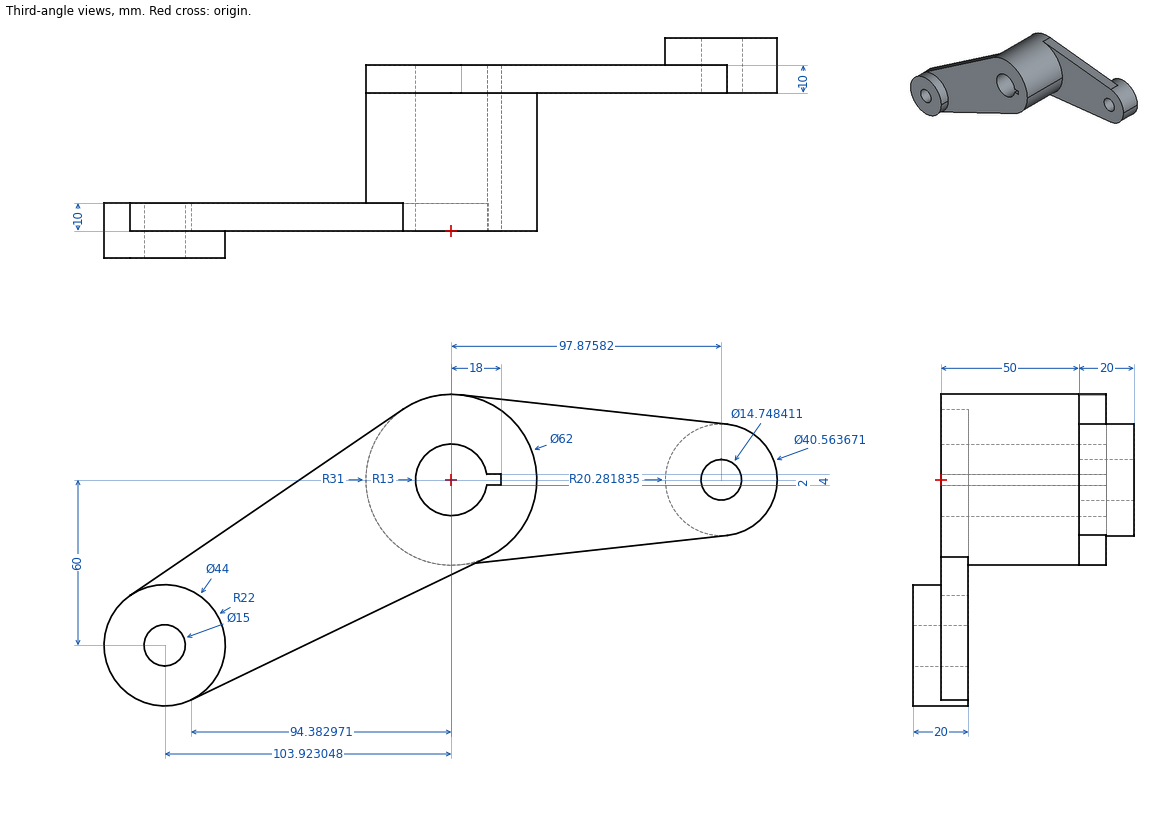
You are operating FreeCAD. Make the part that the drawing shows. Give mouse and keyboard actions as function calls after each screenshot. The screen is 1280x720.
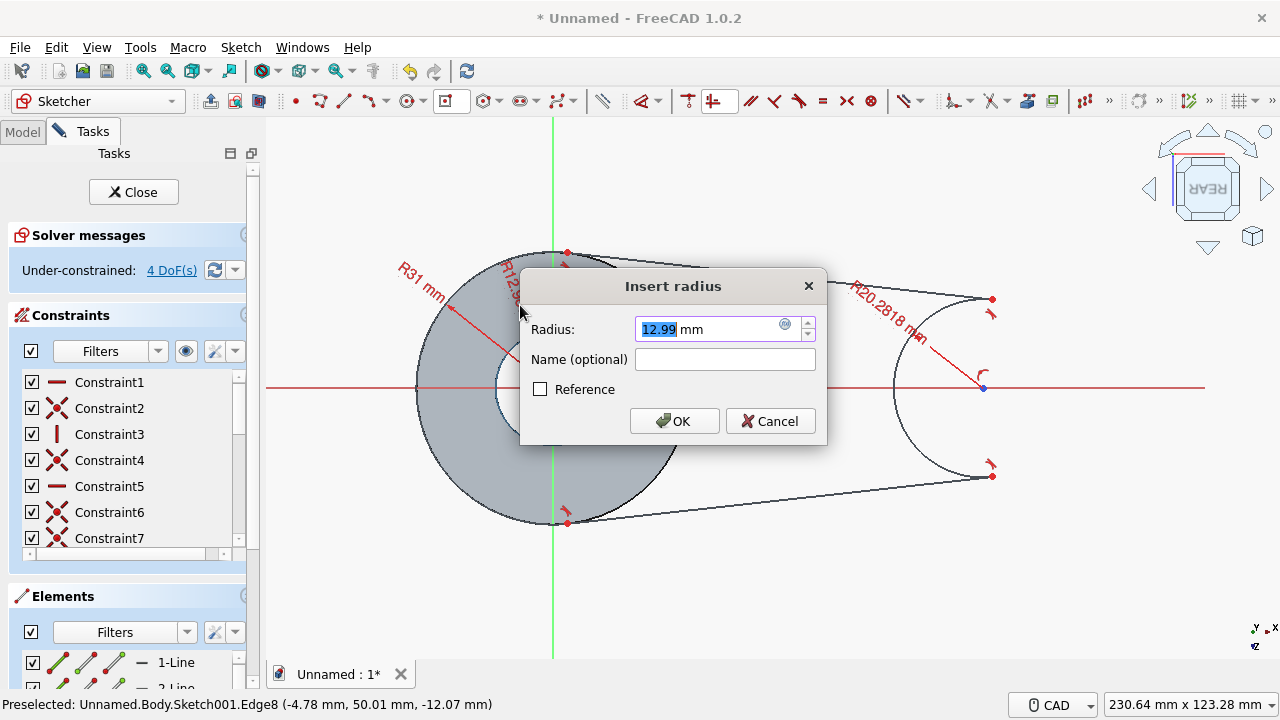
text(13)
key(Return)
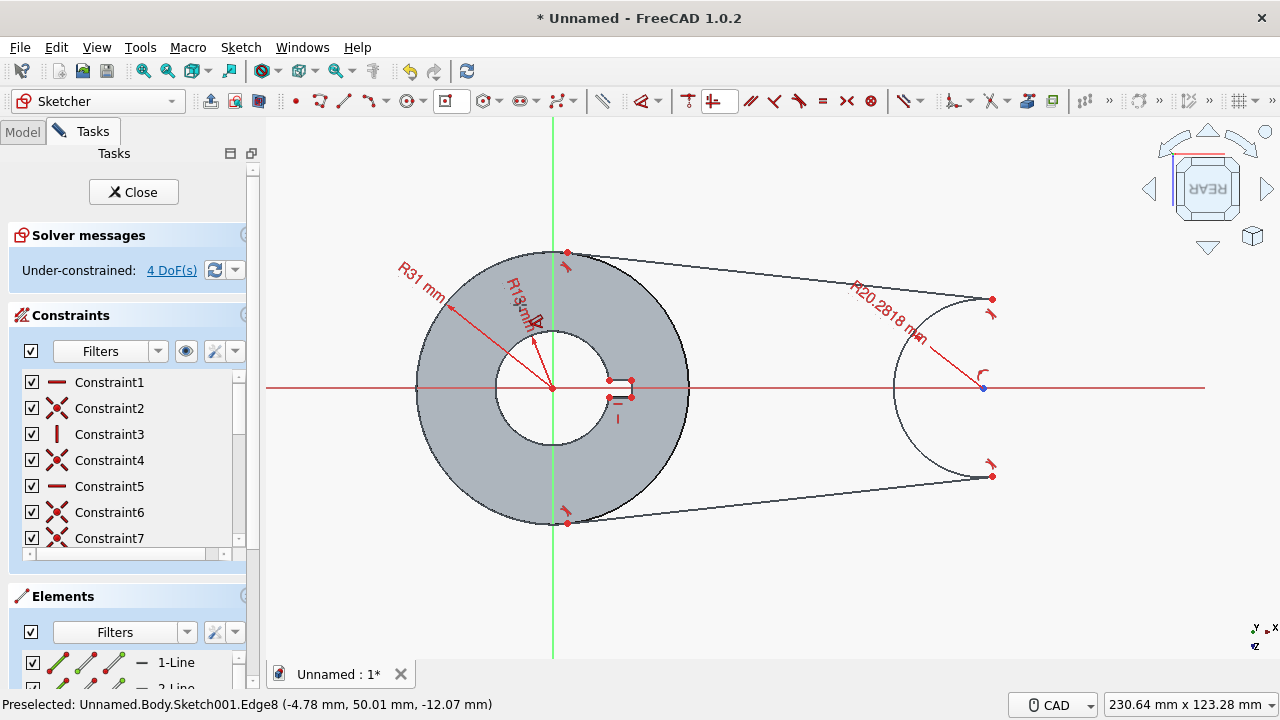
scroll(632, 389, up, 5)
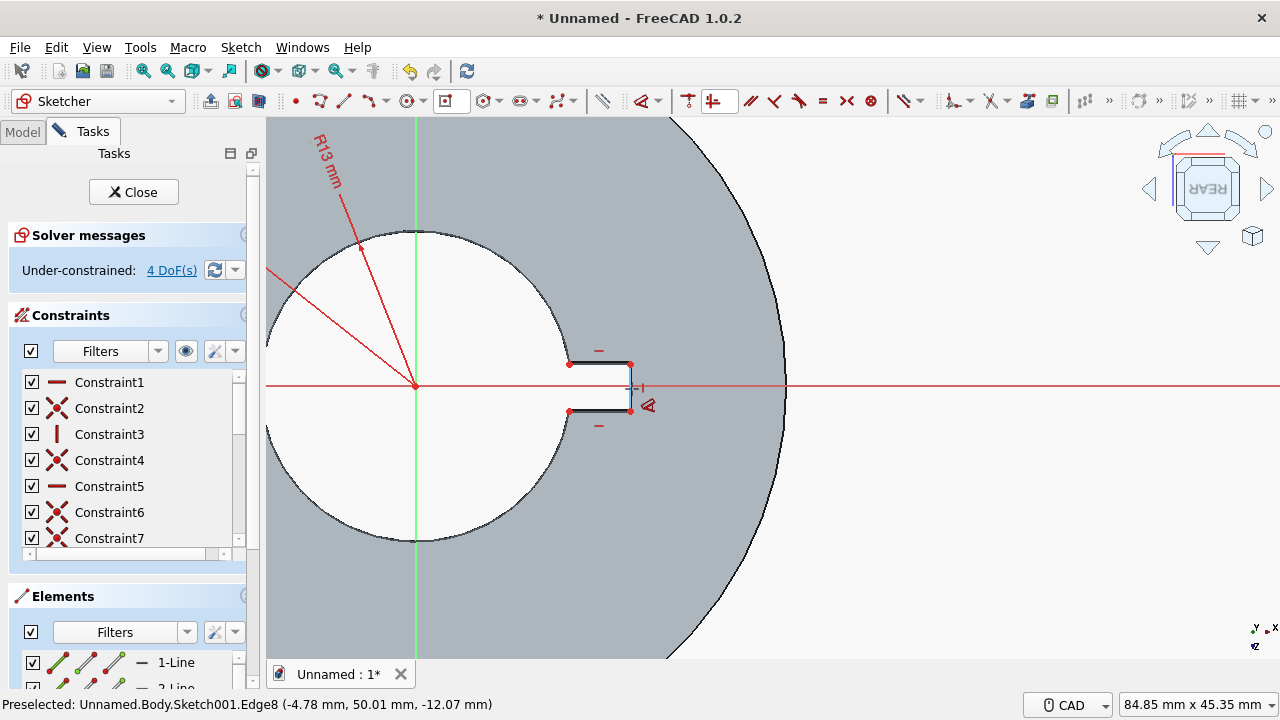
click(630, 388)
click(664, 371)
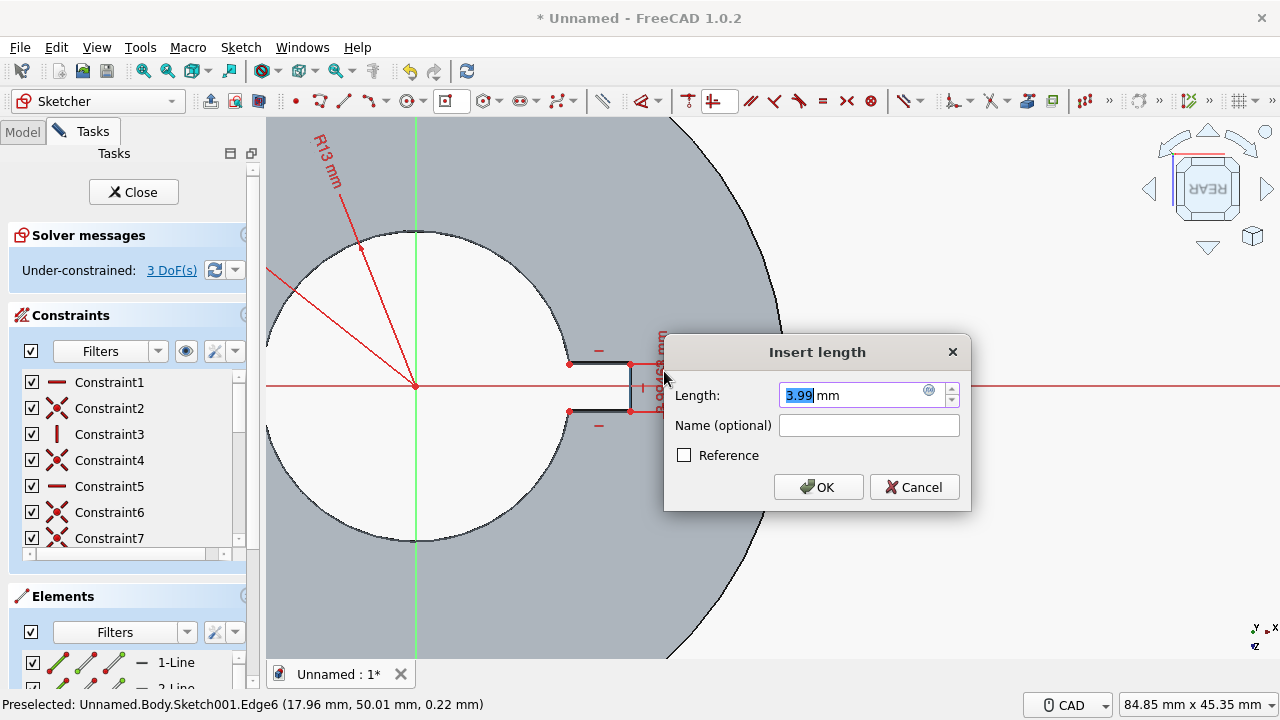
text(4)
key(Return)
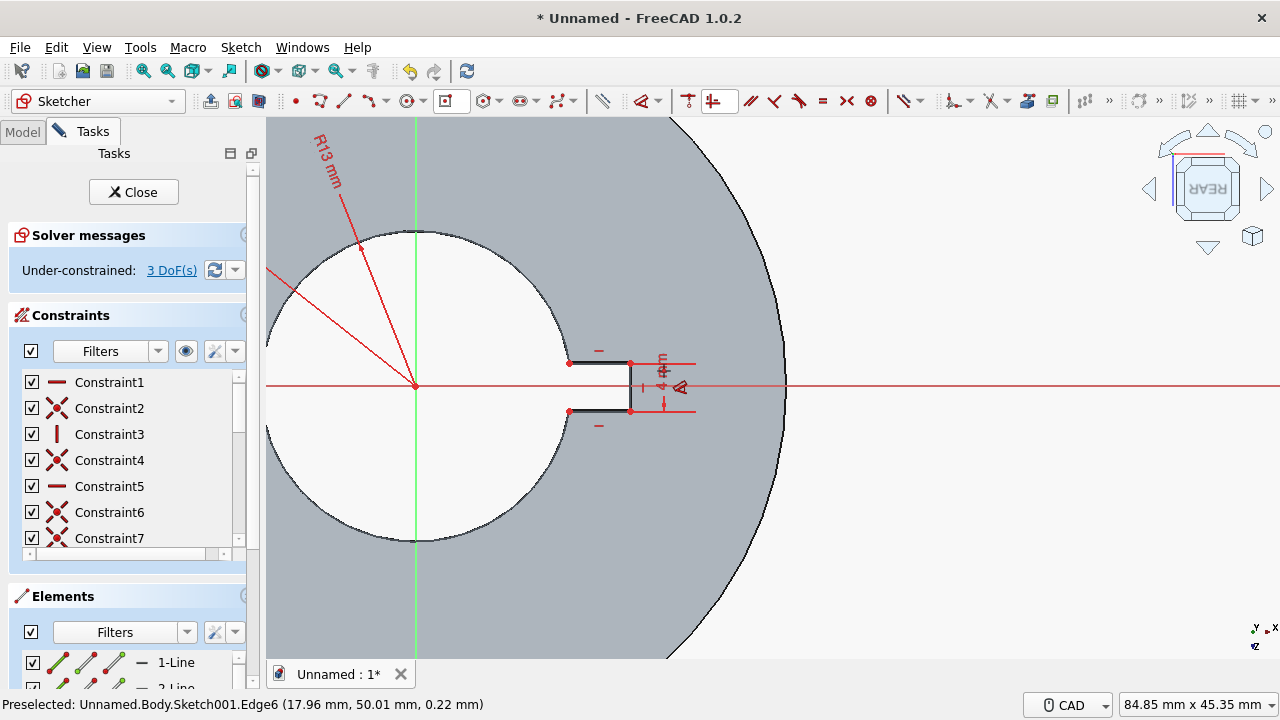
scroll(569, 364, up, 3)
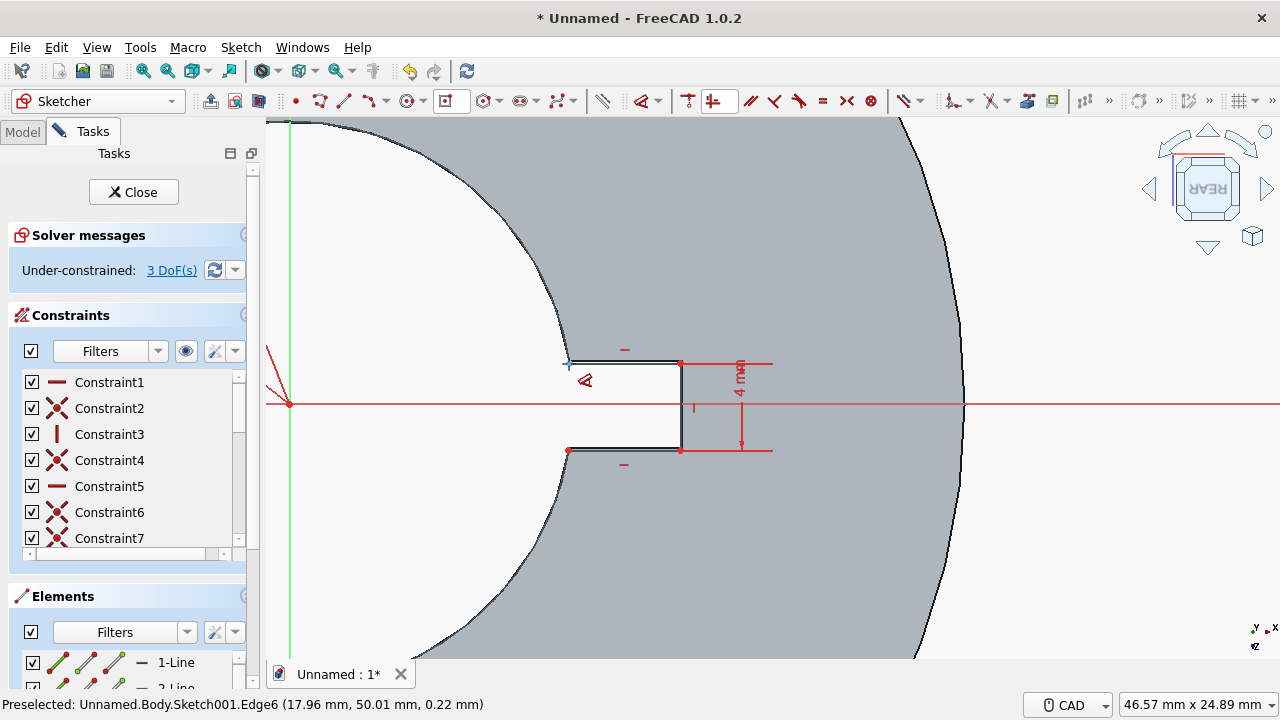
click(570, 364)
click(604, 384)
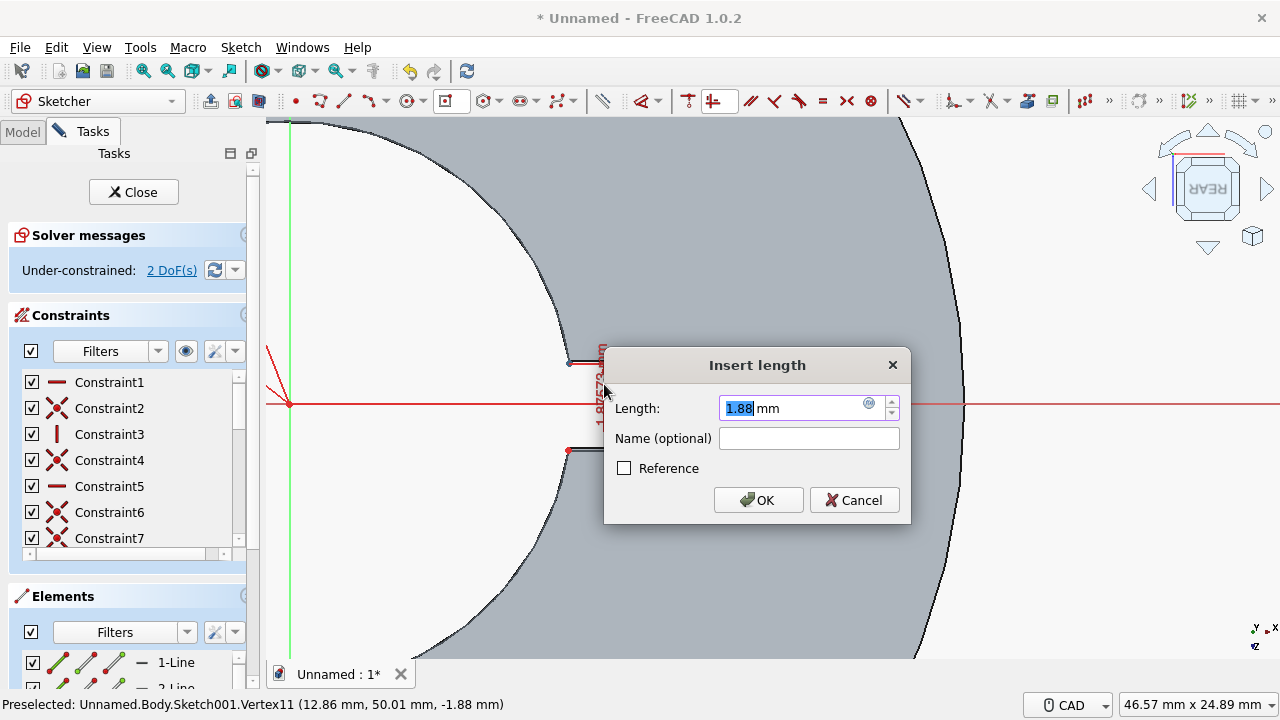
text(2)
key(Return)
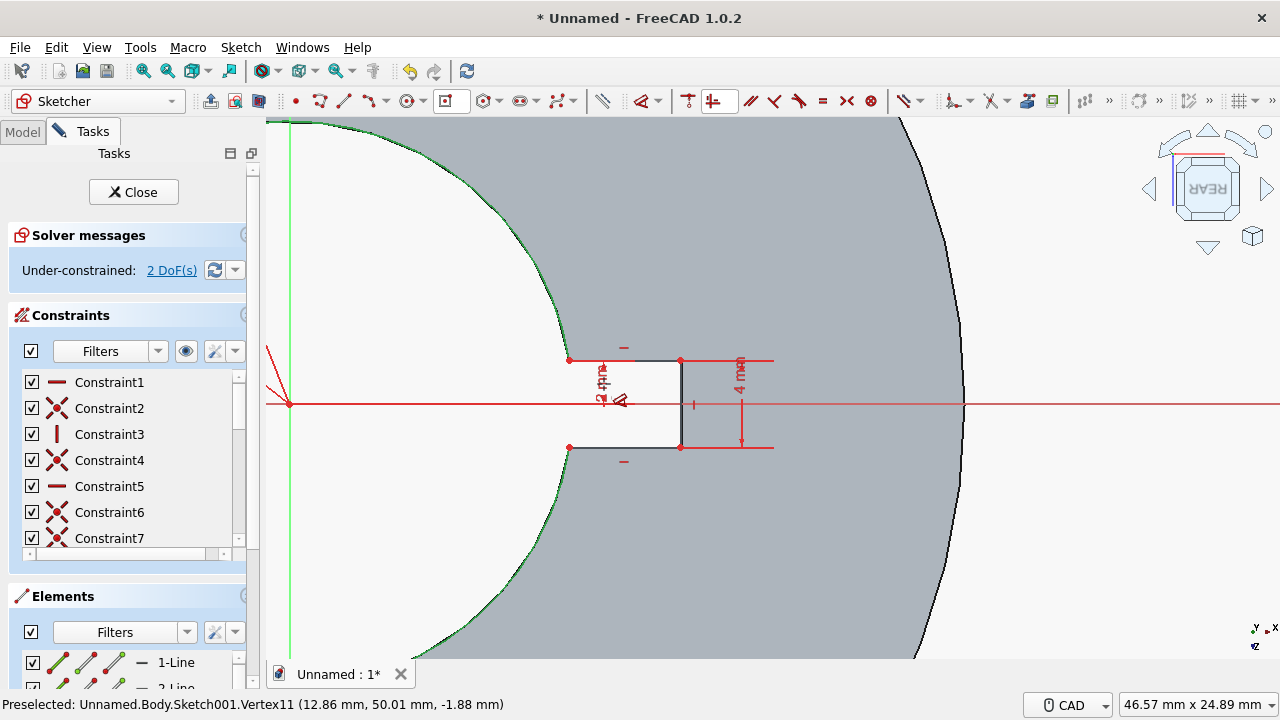
scroll(619, 384, down, 8)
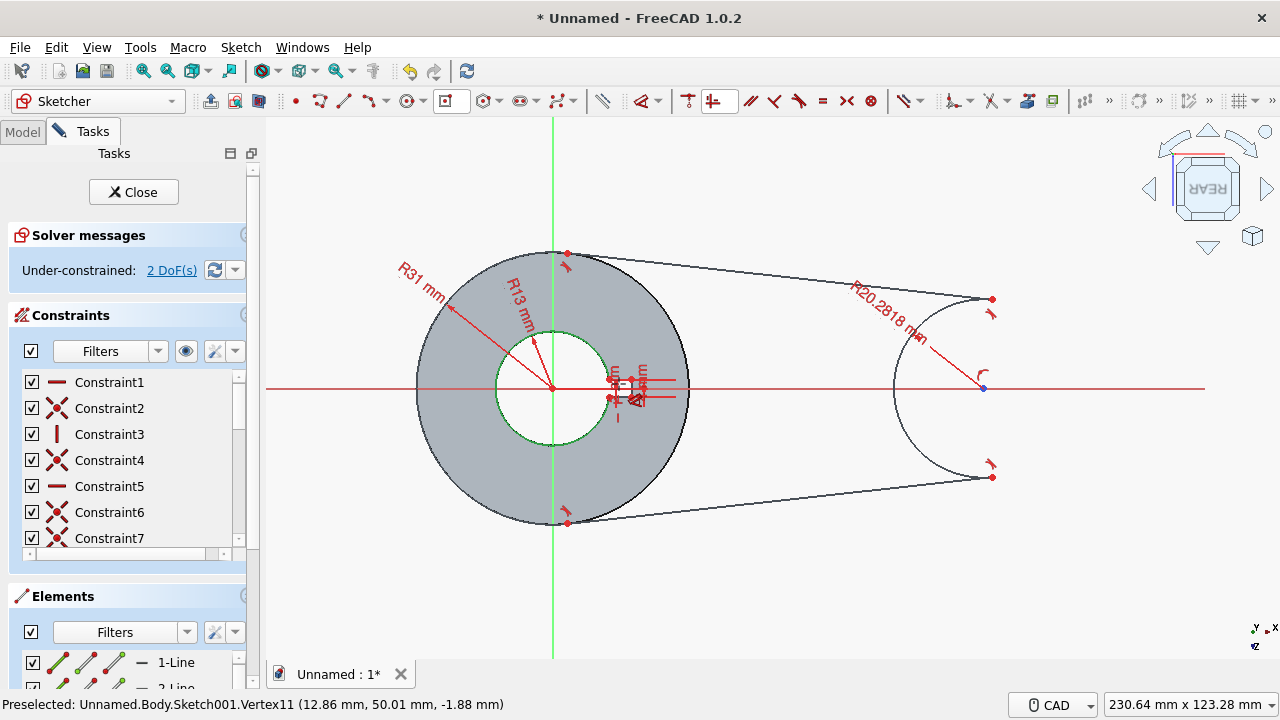
click(632, 380)
click(610, 346)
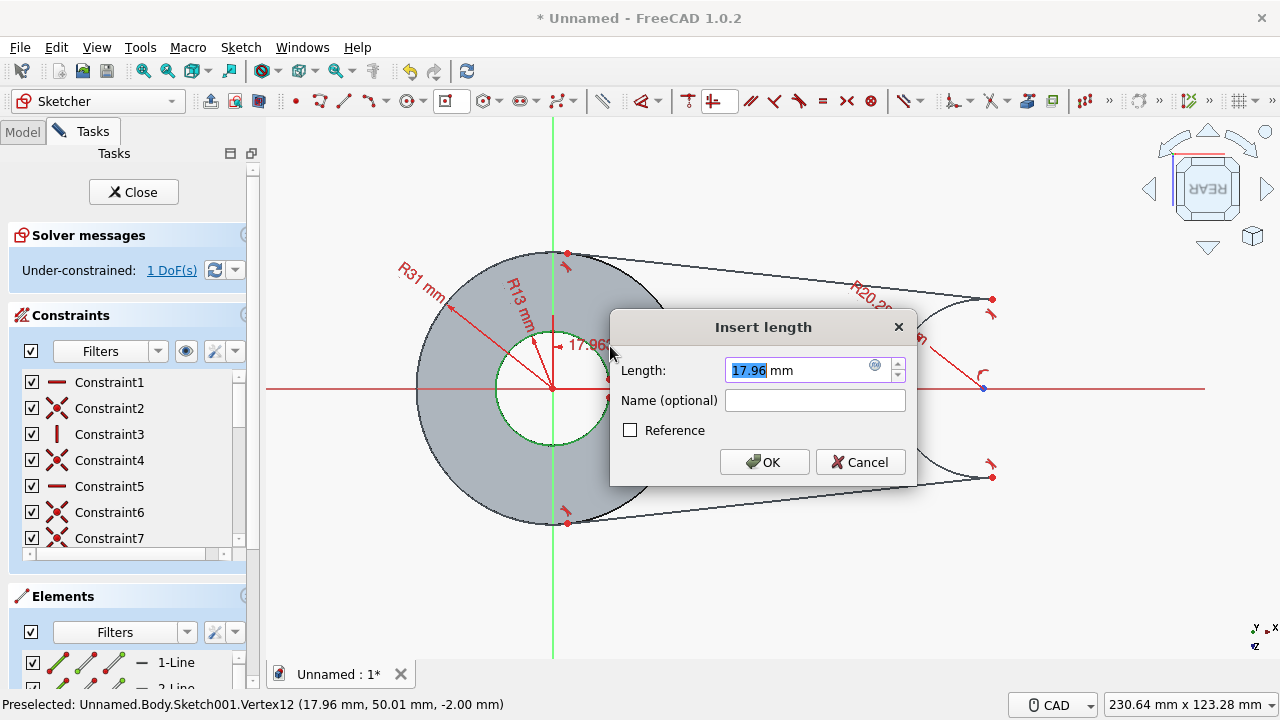
text(18)
key(Return)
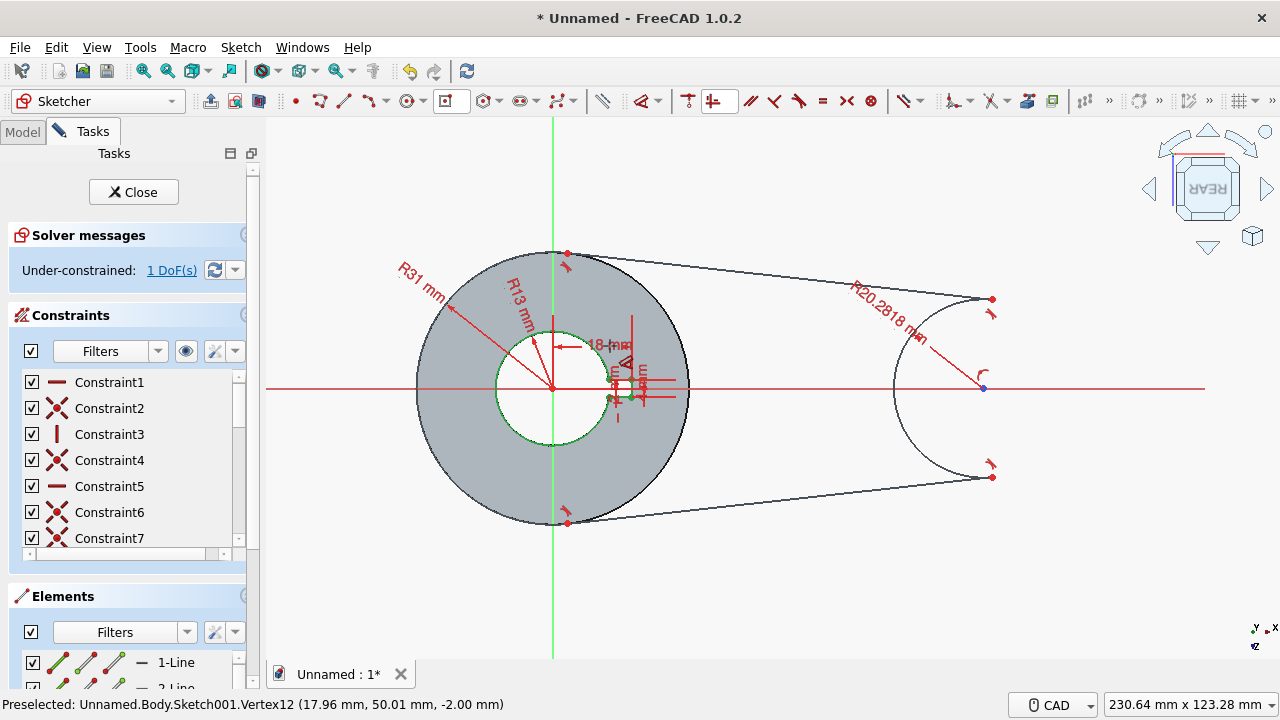
click(983, 389)
click(768, 423)